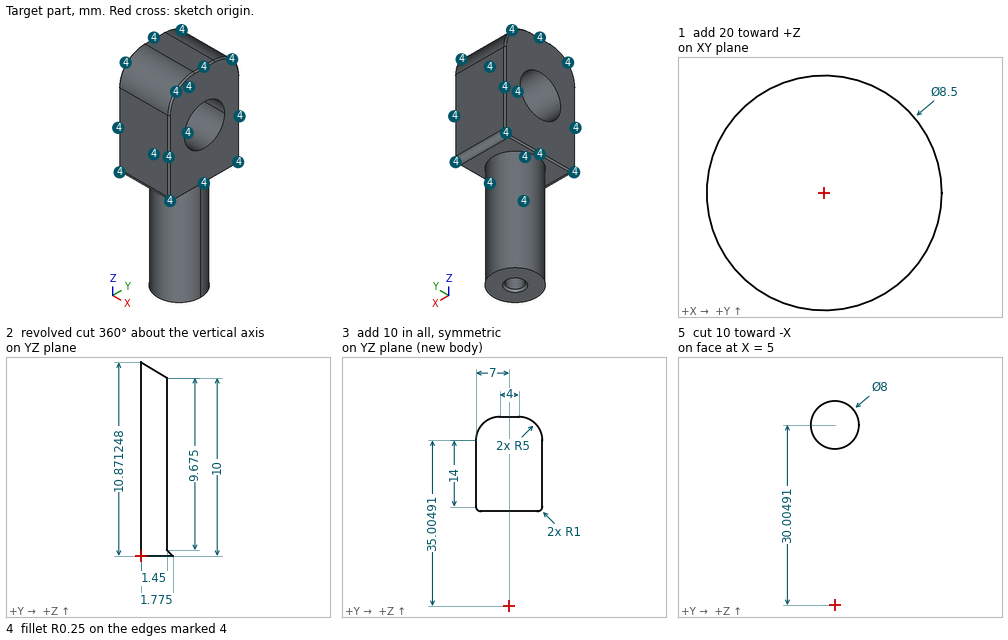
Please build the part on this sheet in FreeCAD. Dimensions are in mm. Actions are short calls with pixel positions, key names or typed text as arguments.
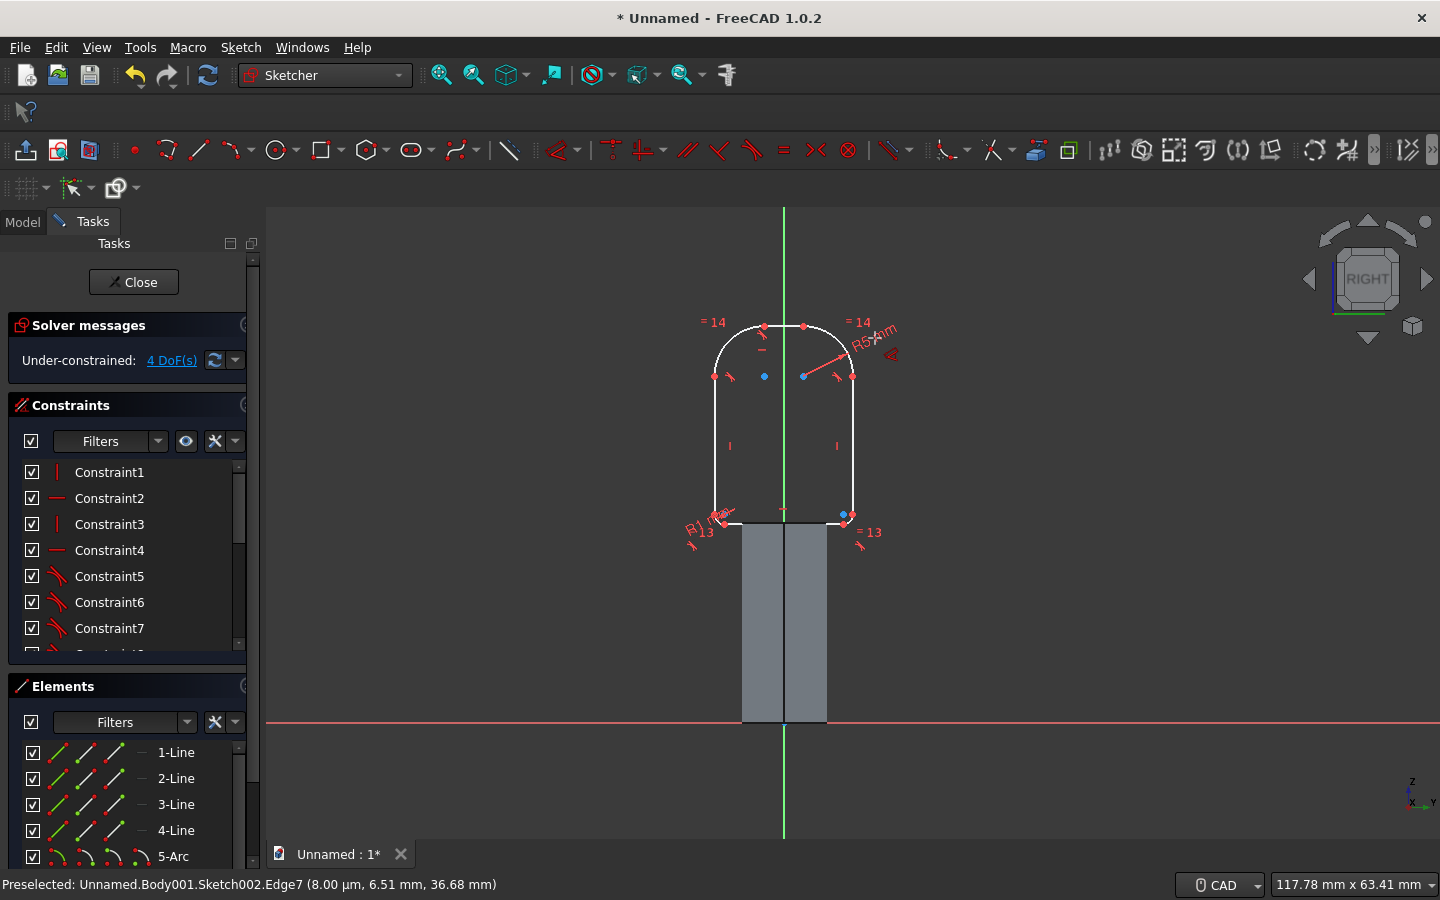
click(788, 326)
click(770, 292)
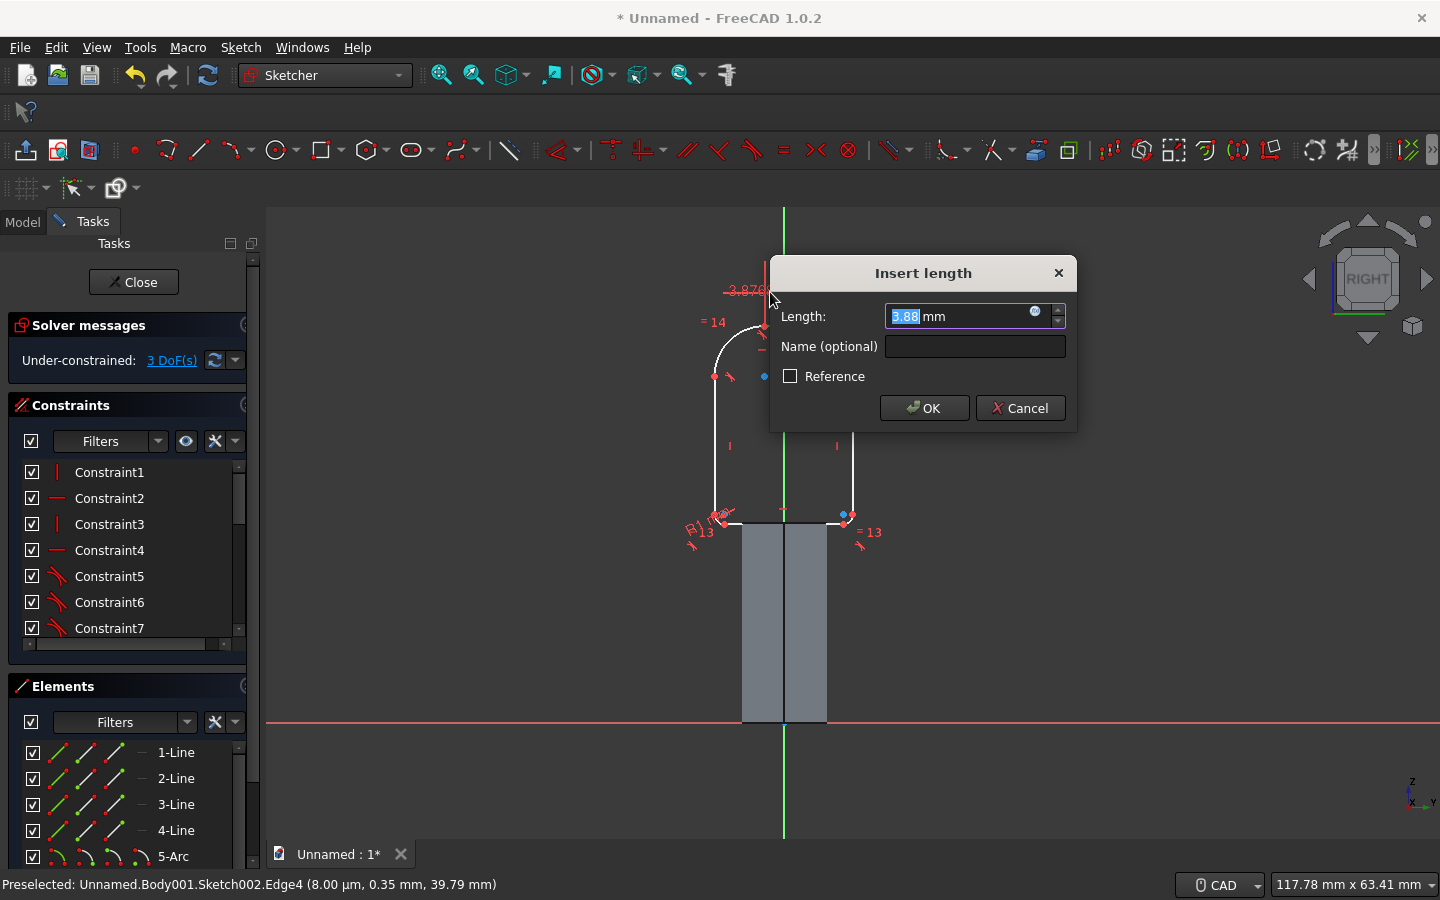
text(4)
key(Return)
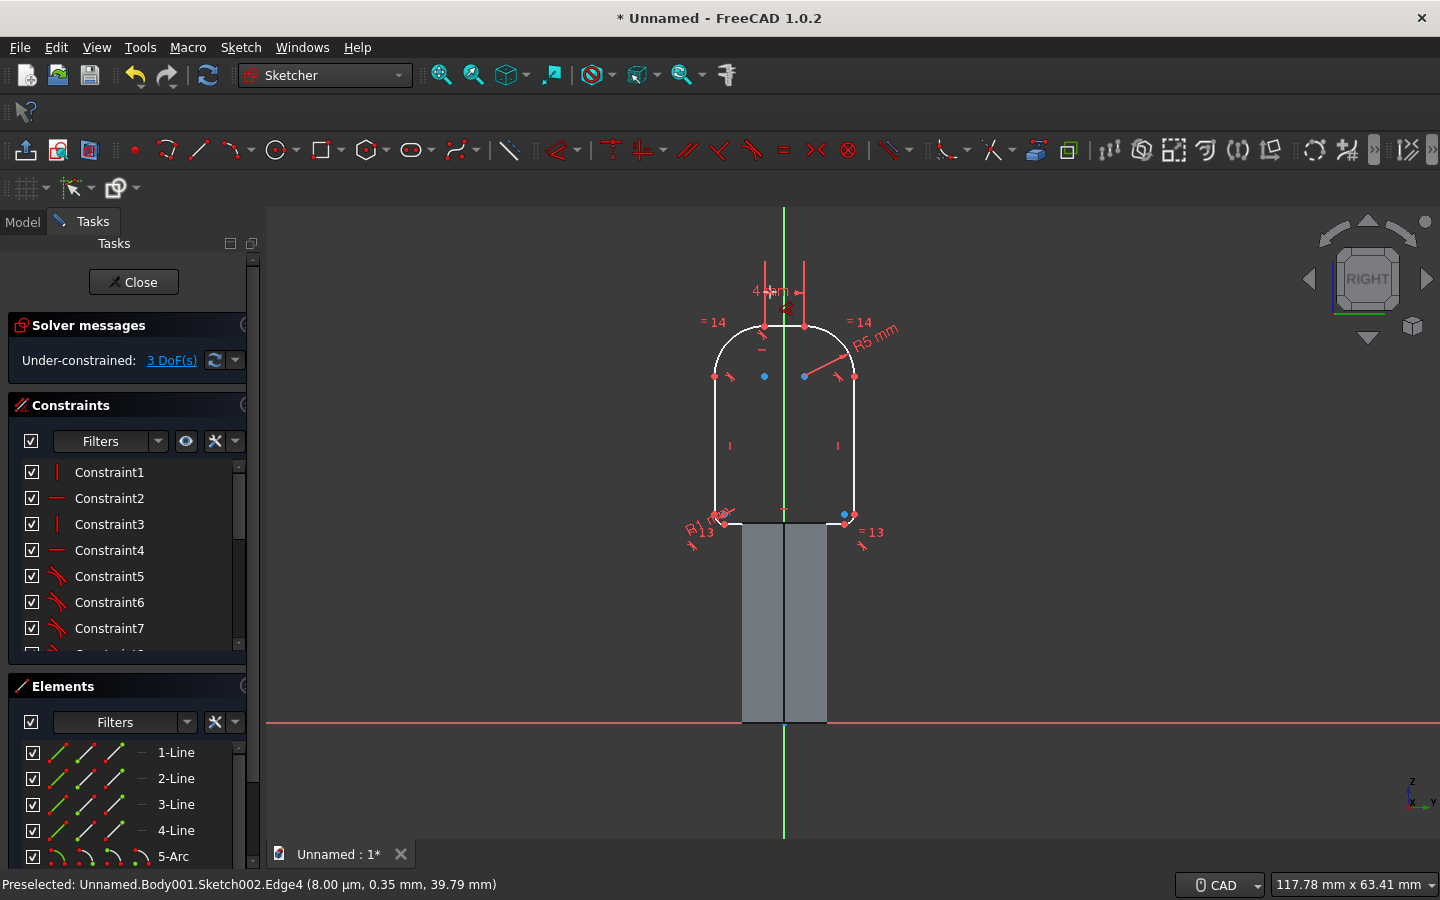
click(715, 418)
click(681, 445)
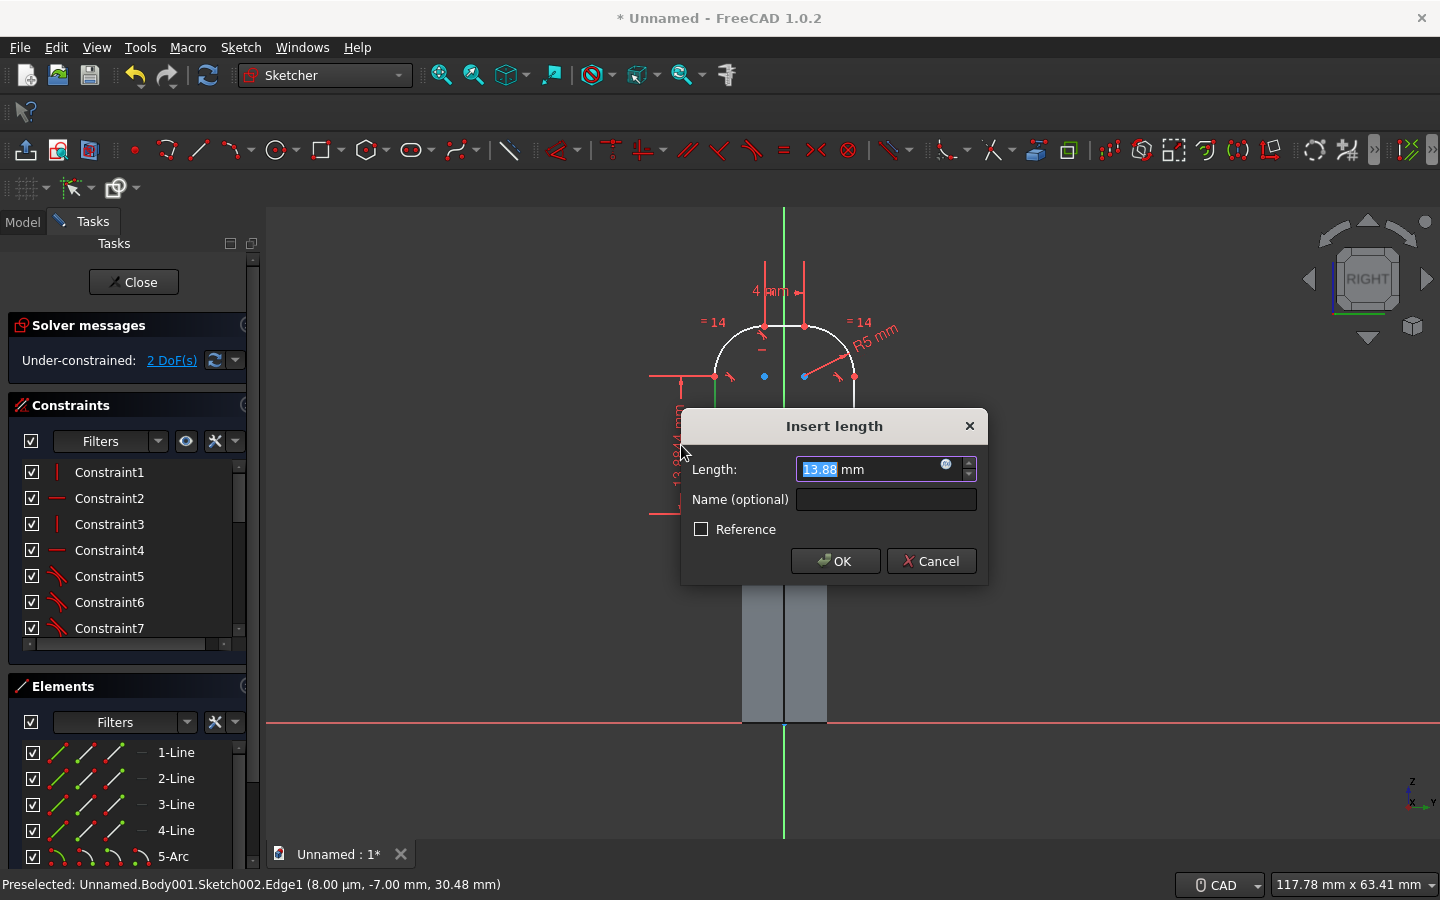
text(14)
key(Return)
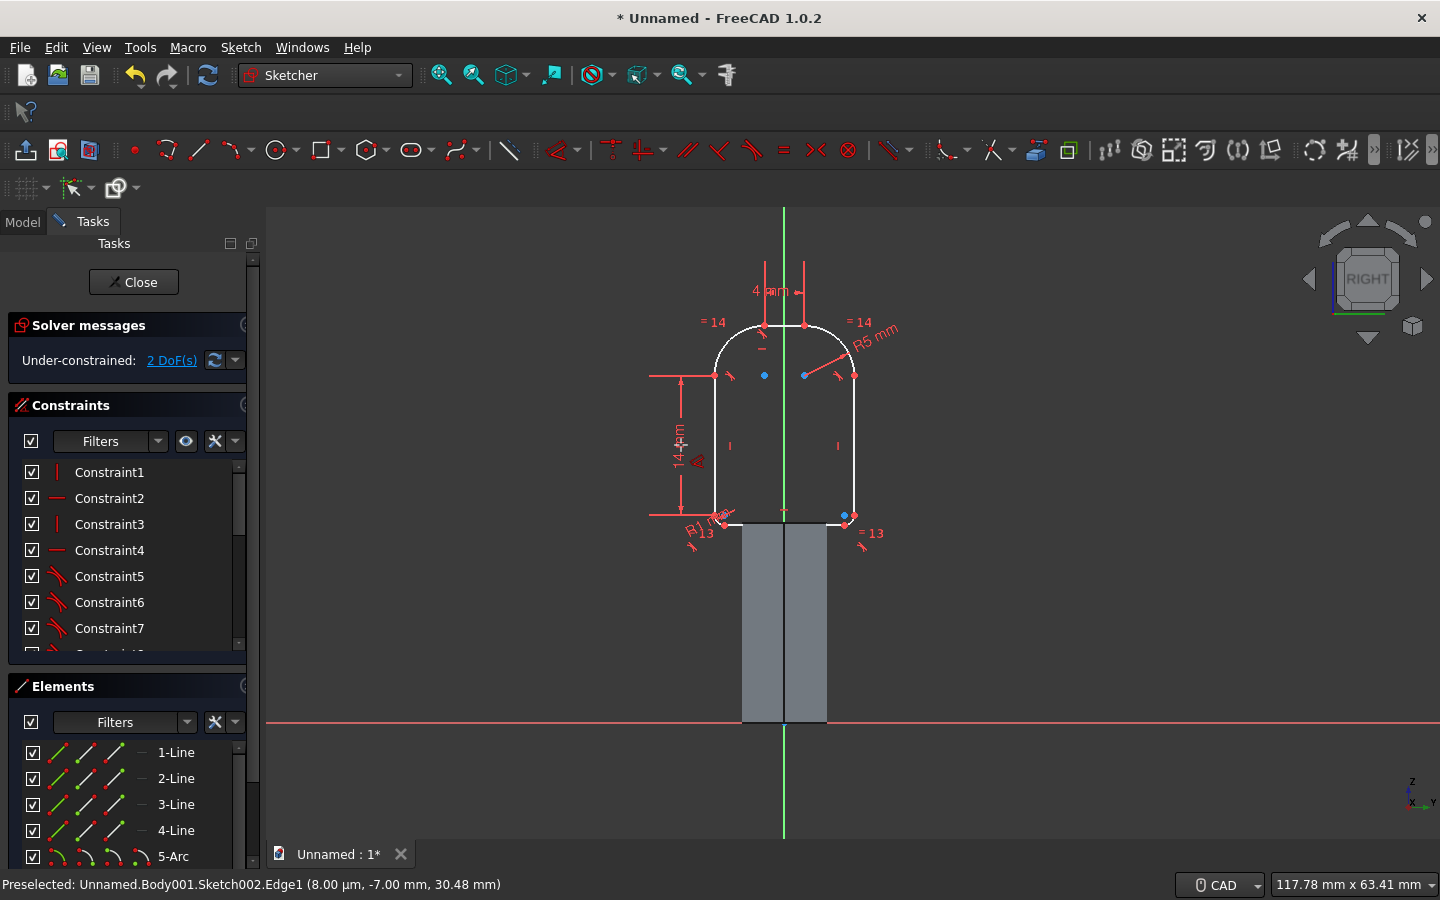
click(715, 376)
click(750, 757)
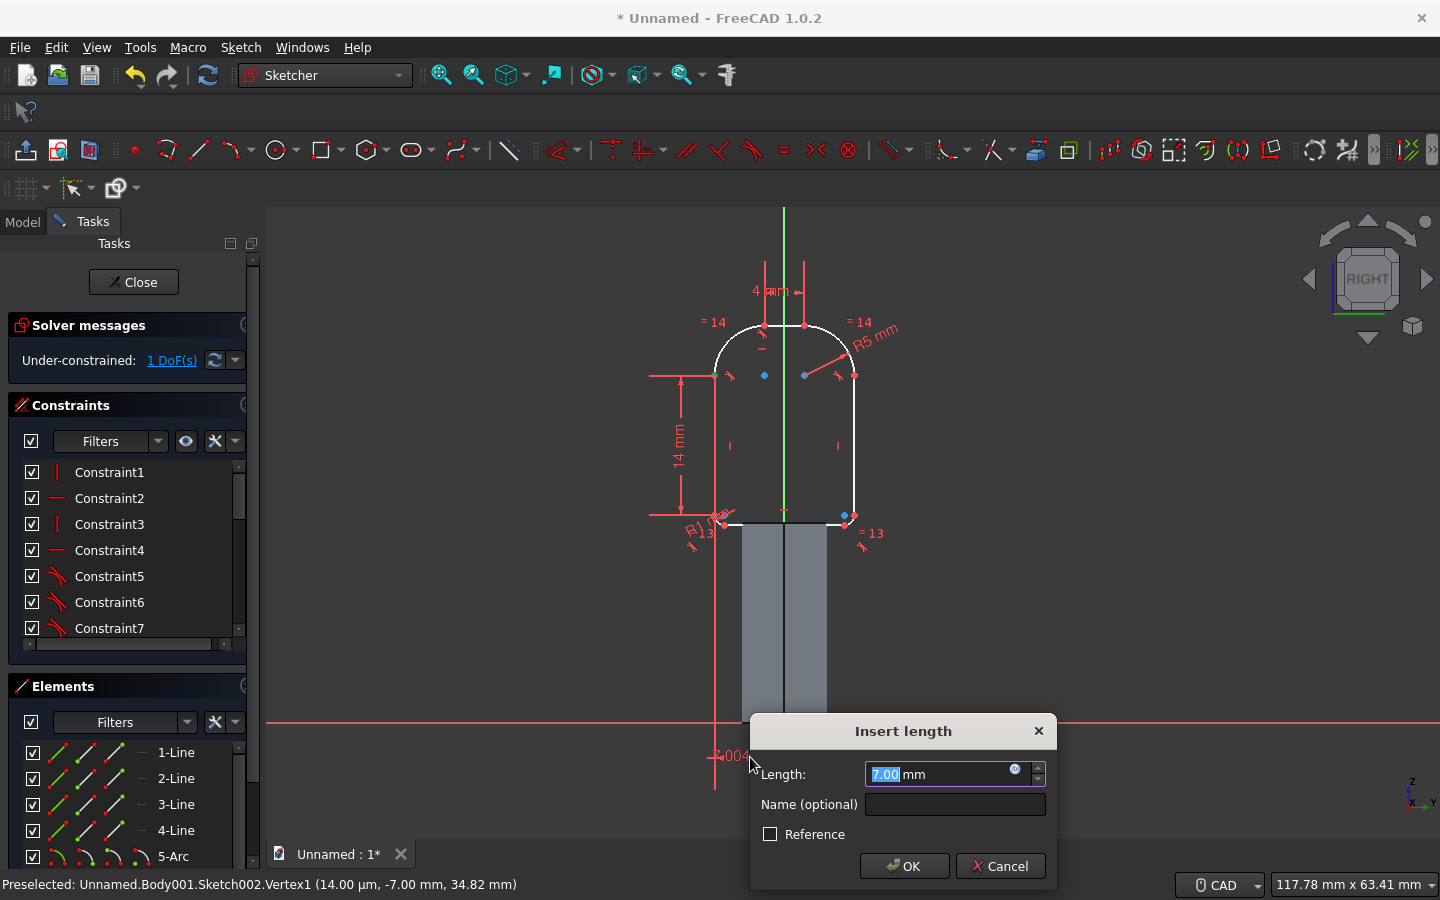
text(7)
key(Return)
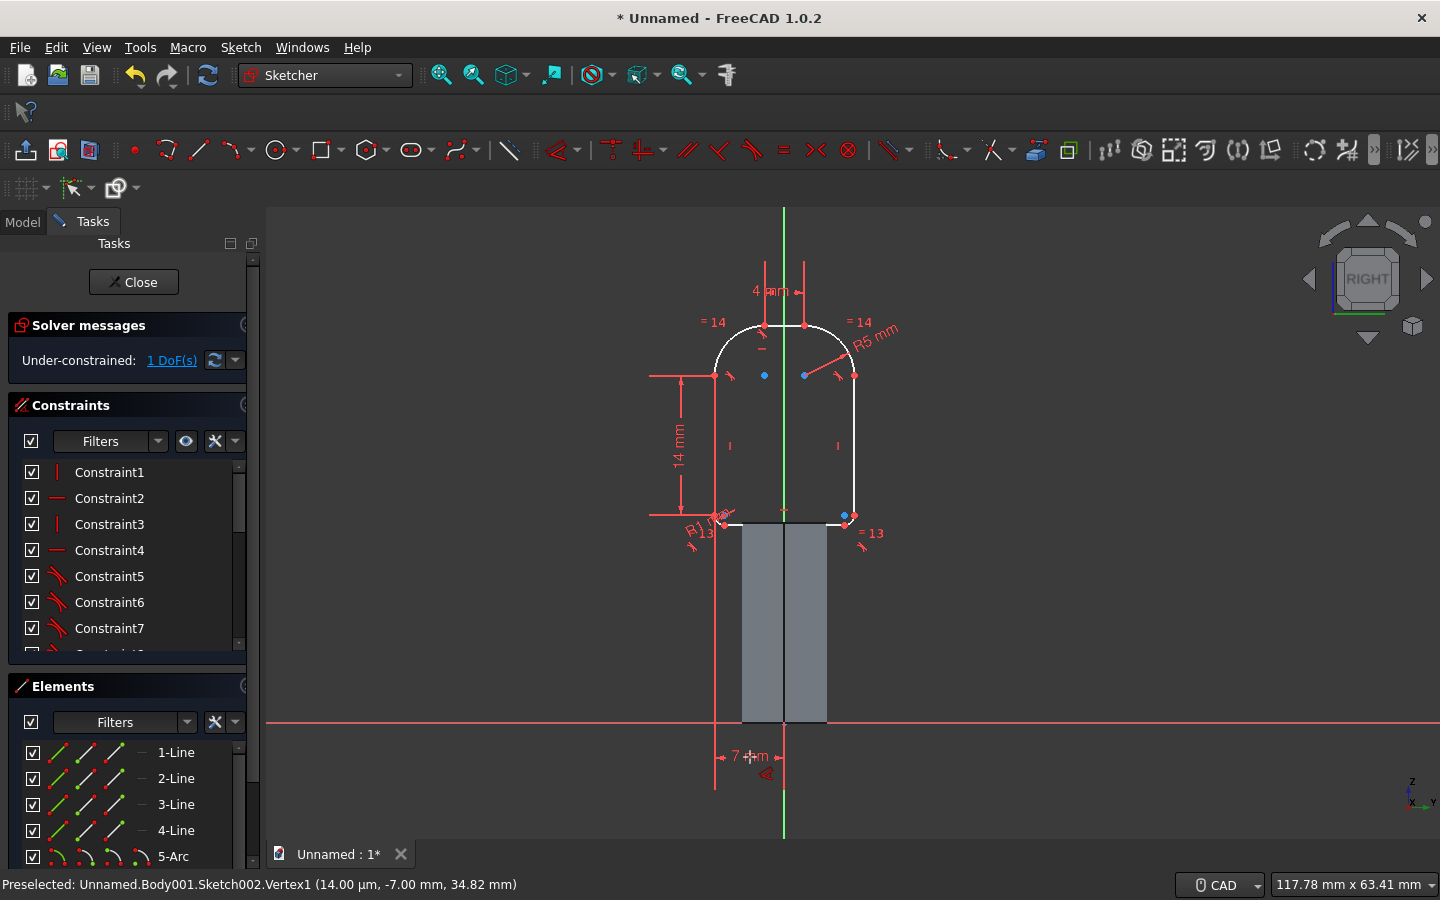
click(715, 376)
click(681, 549)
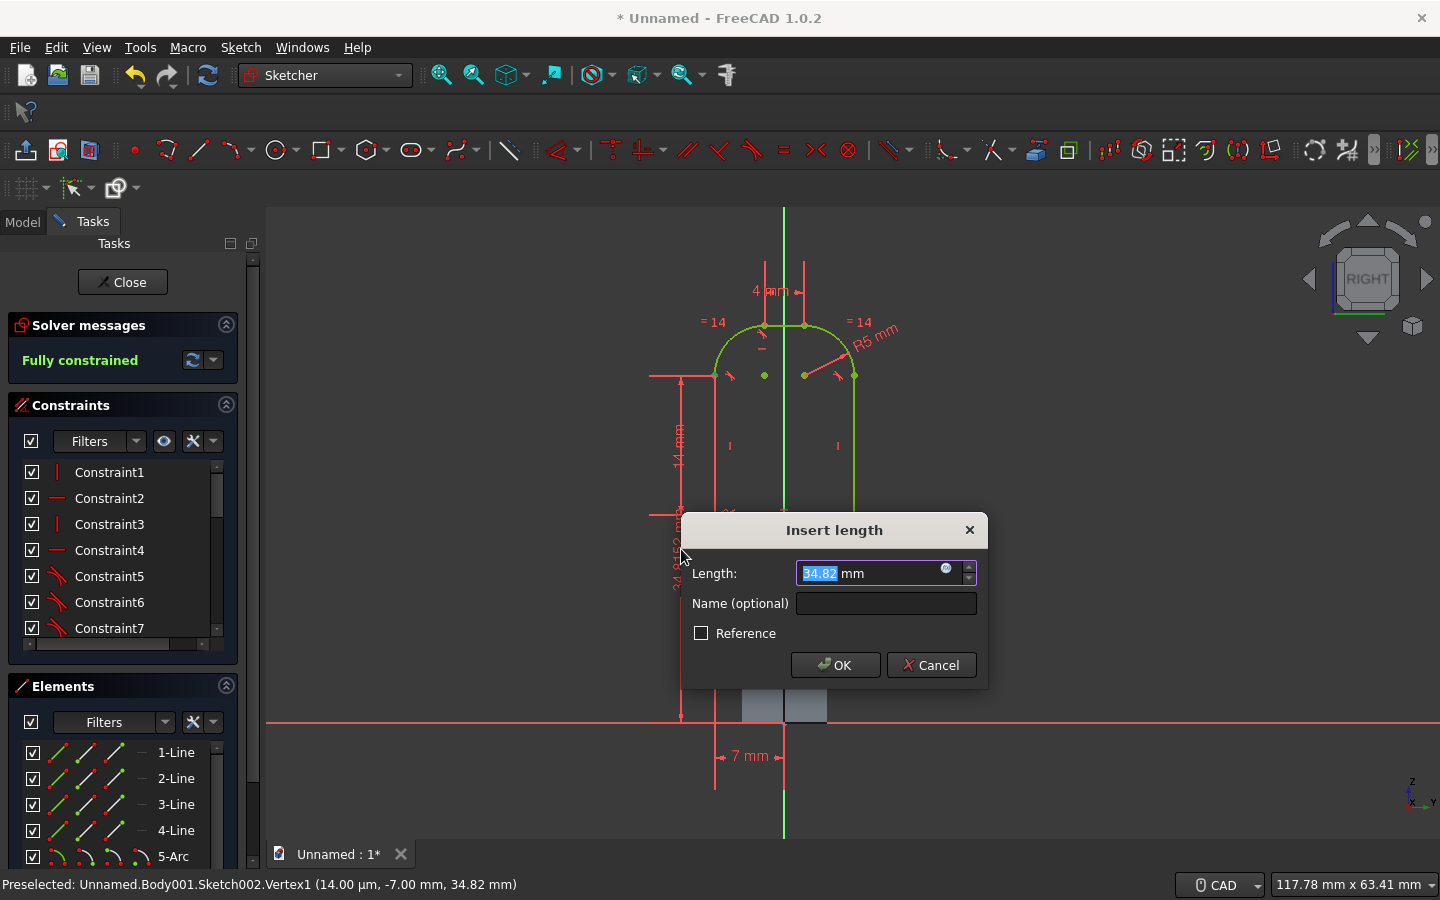
text(35.00491)
key(Return)
key(Escape)